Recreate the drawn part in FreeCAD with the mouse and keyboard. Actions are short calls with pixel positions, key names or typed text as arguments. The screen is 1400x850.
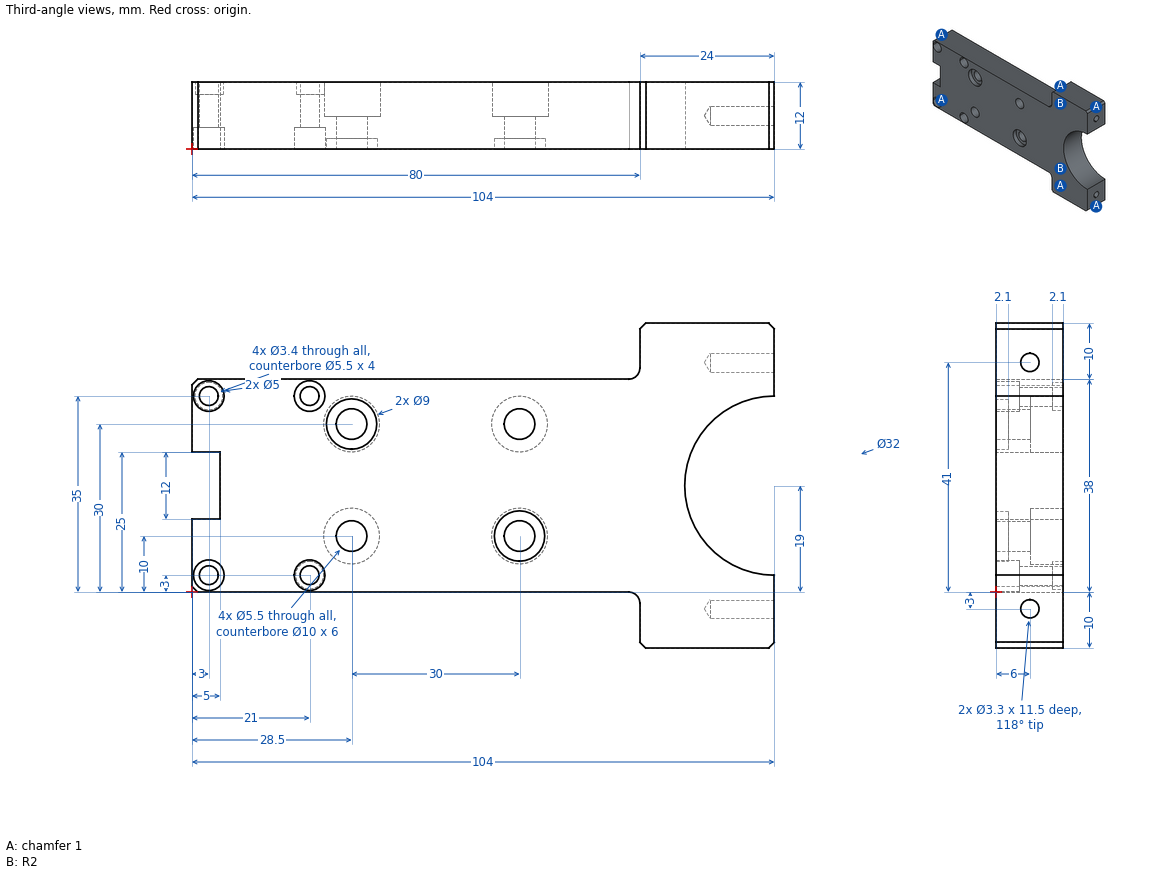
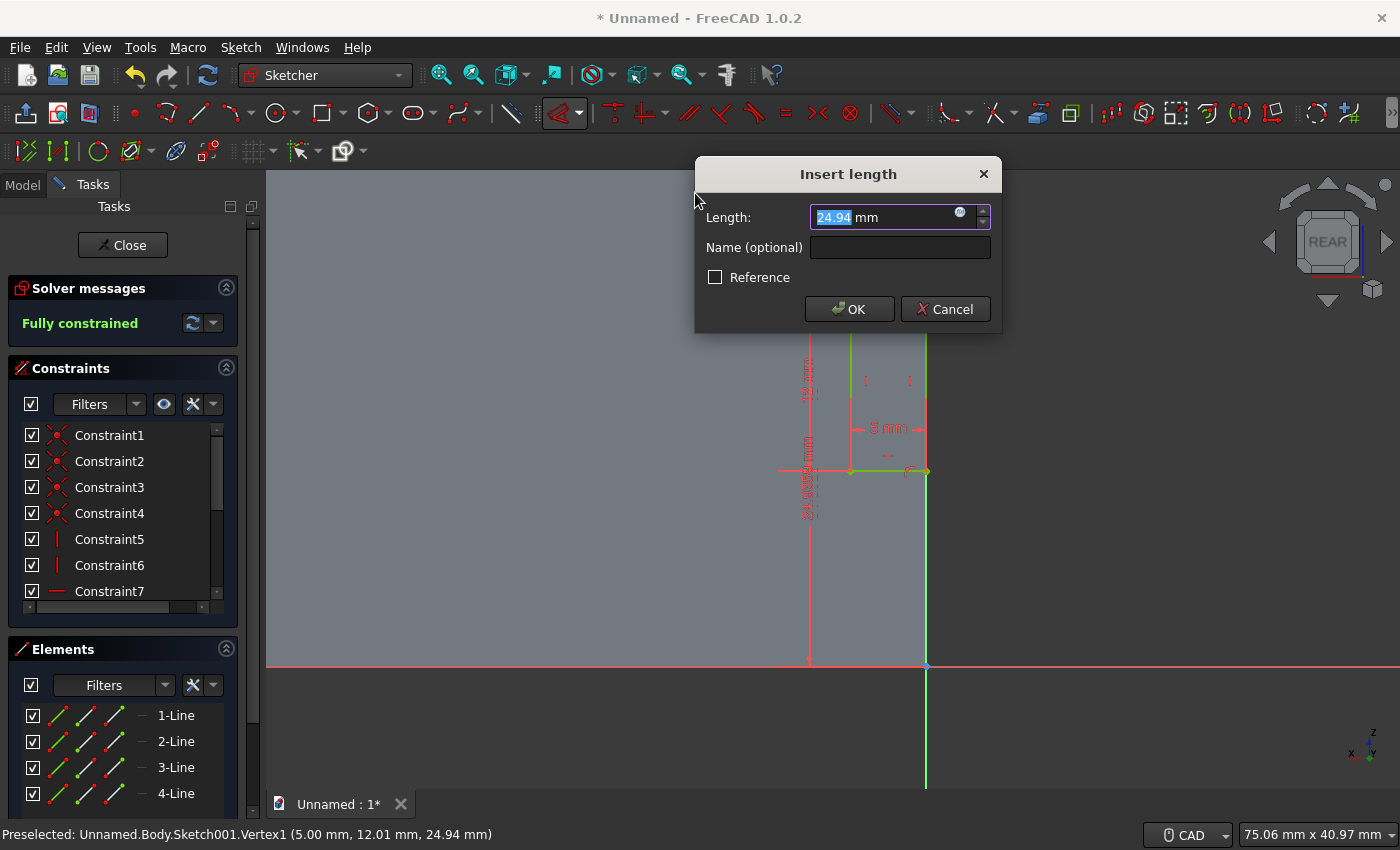
text(25)
key(Return)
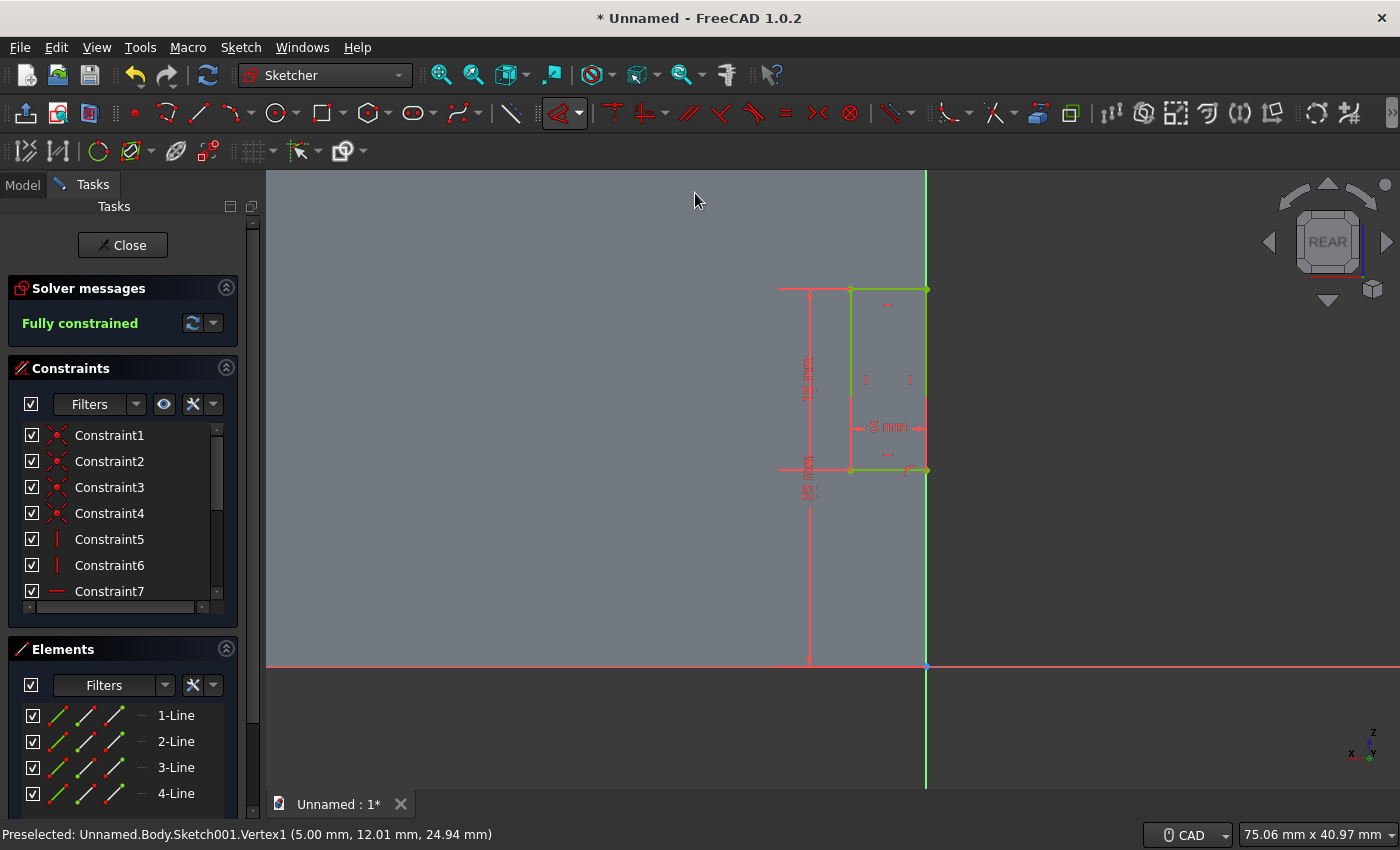
click(123, 245)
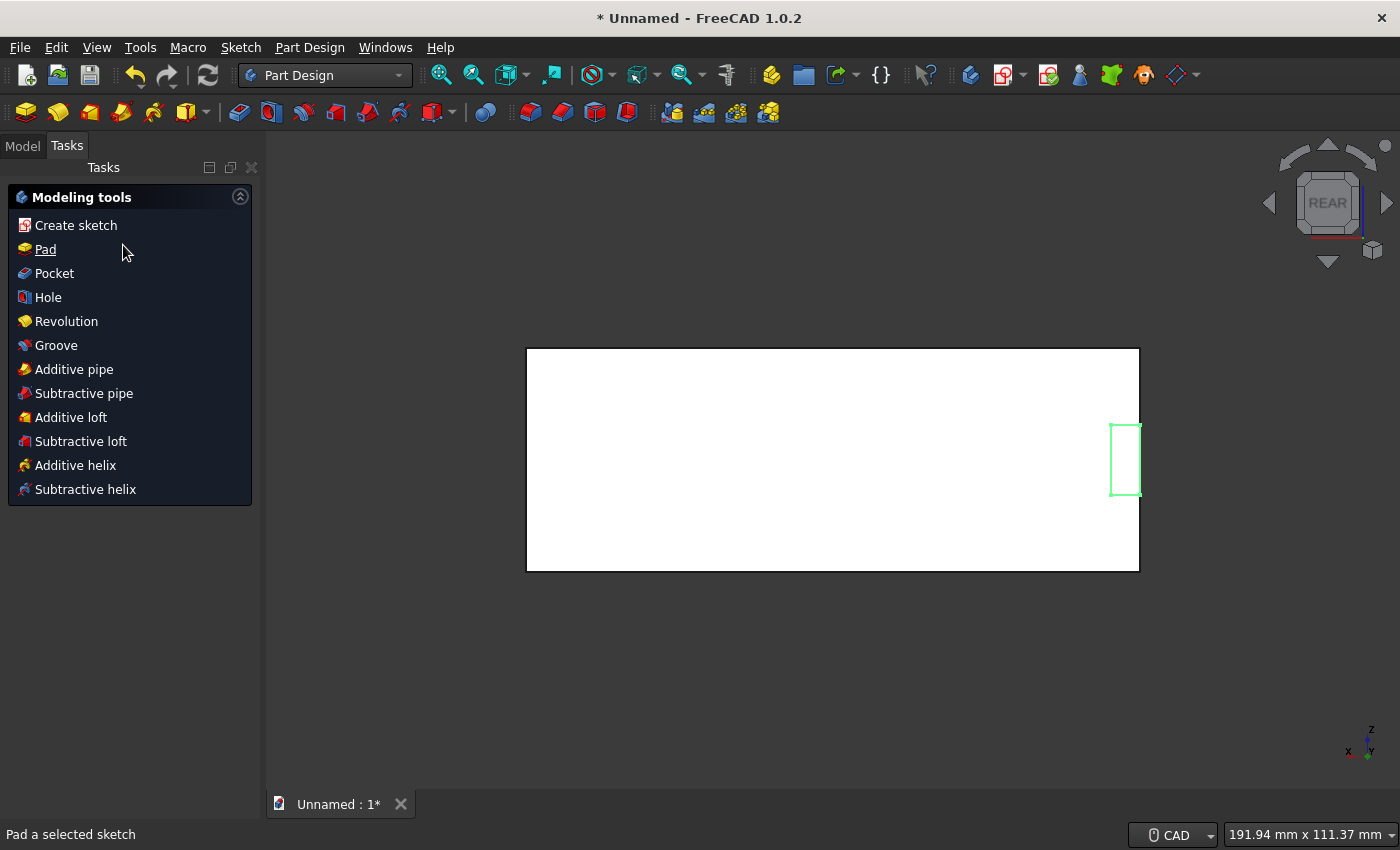
click(240, 112)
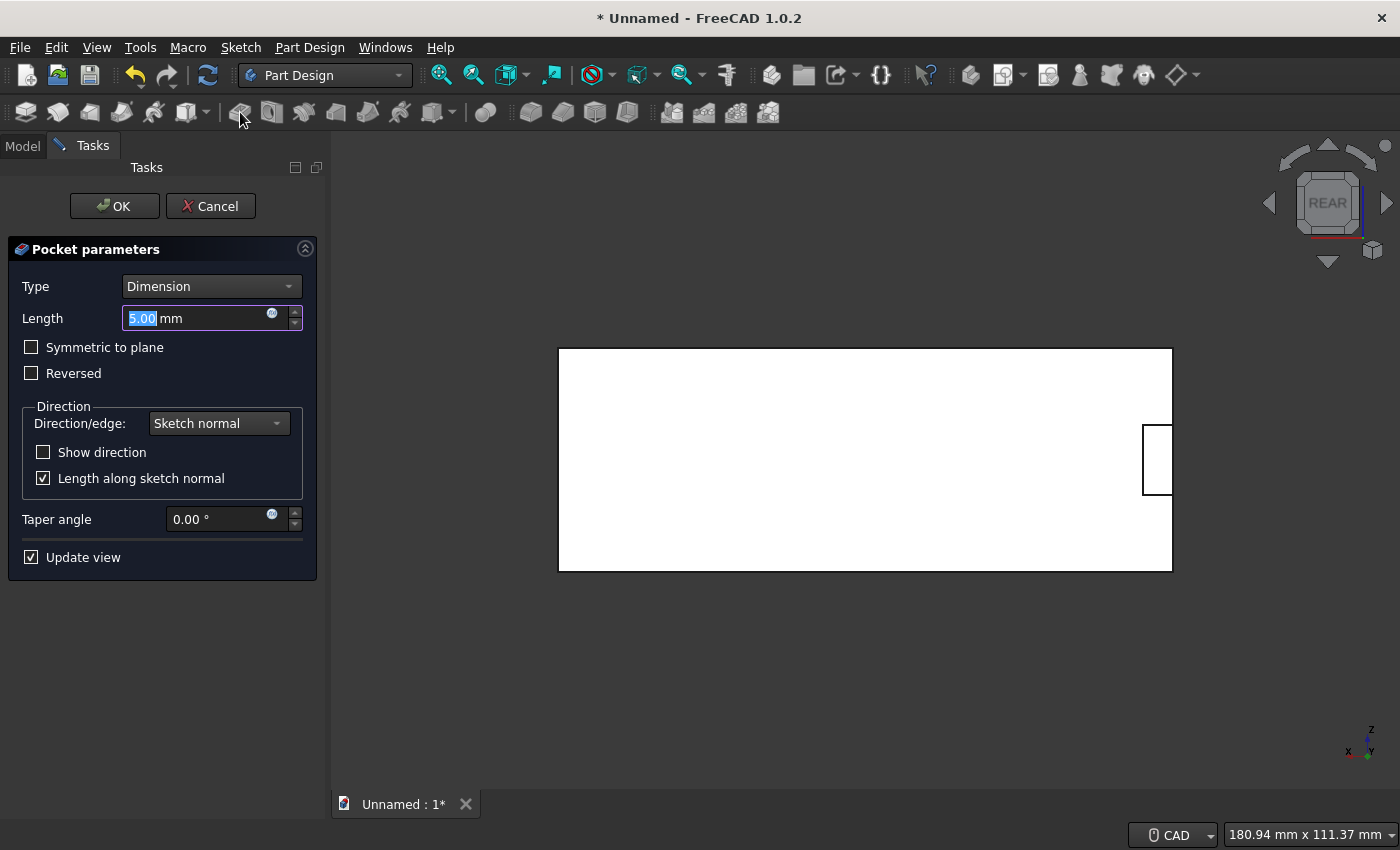
click(212, 286)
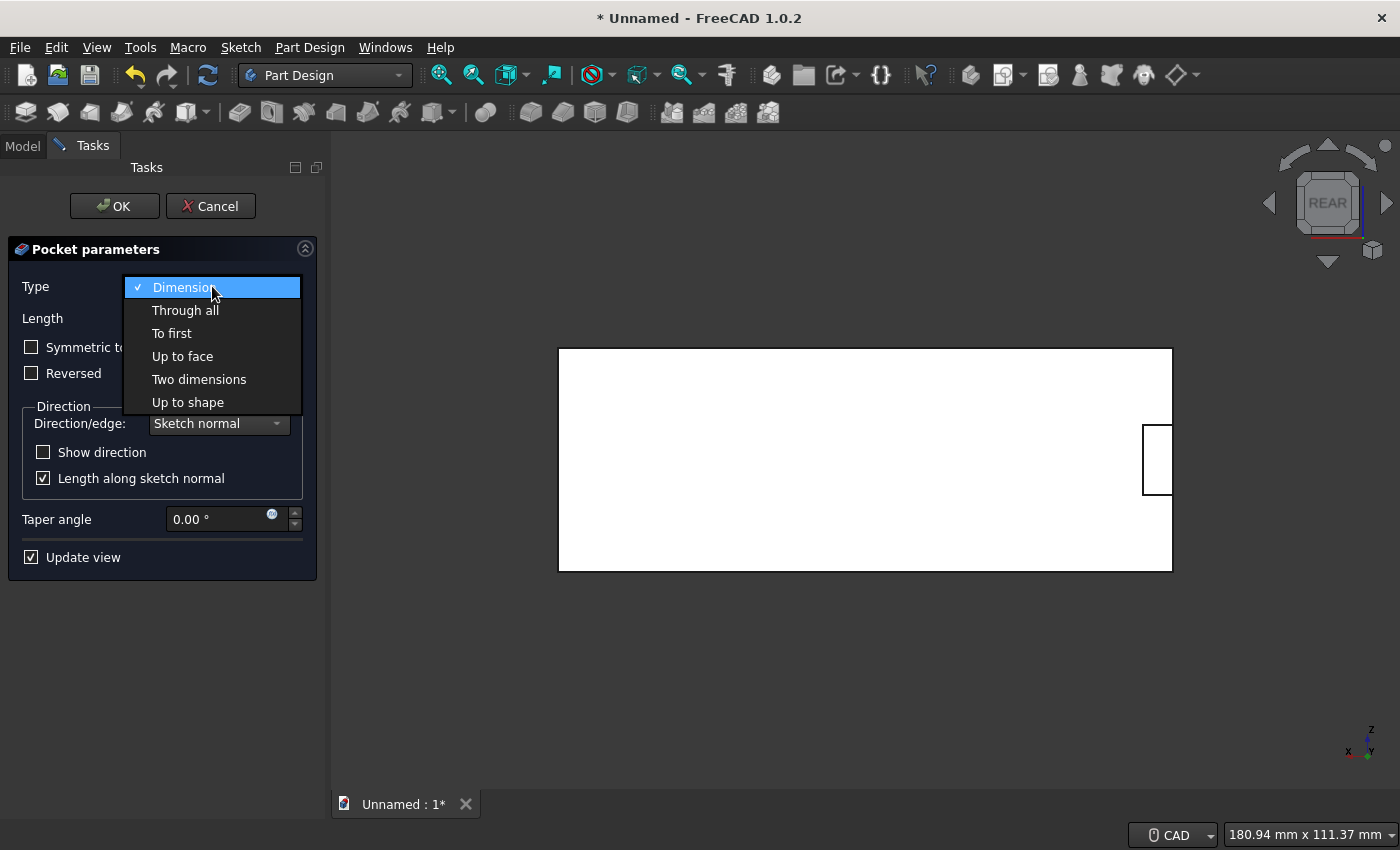
click(212, 310)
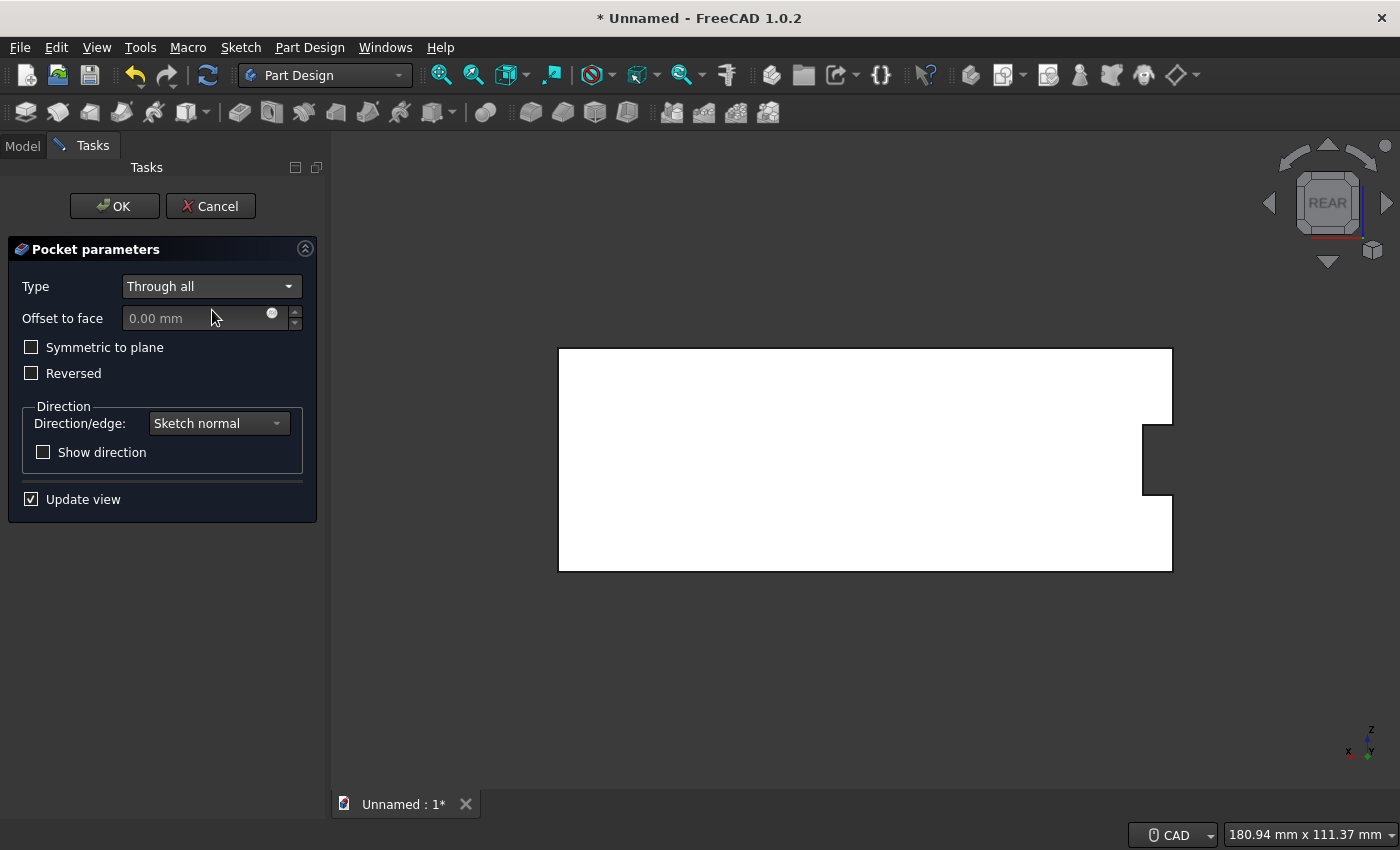
click(115, 206)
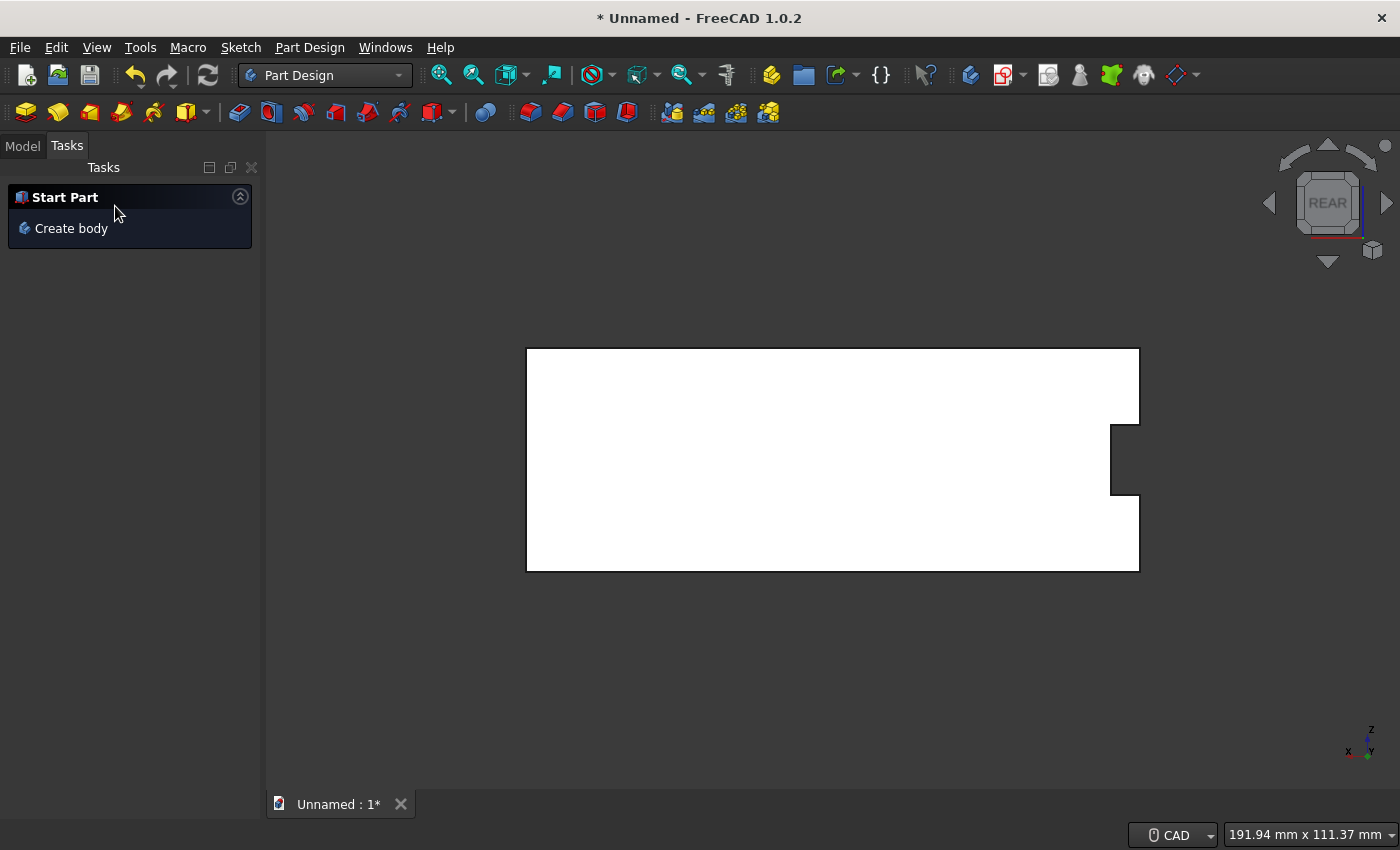
click(657, 459)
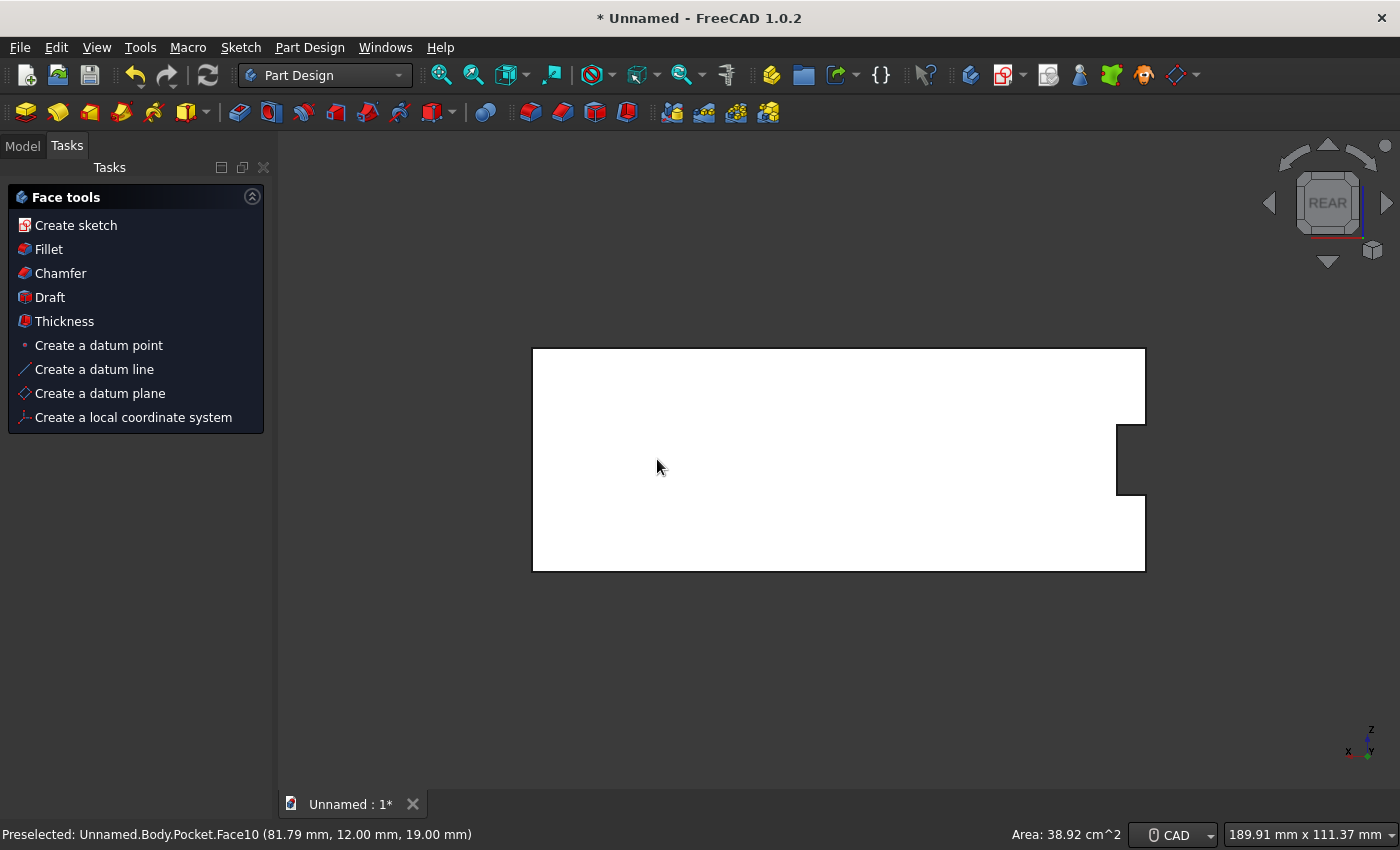
click(1004, 76)